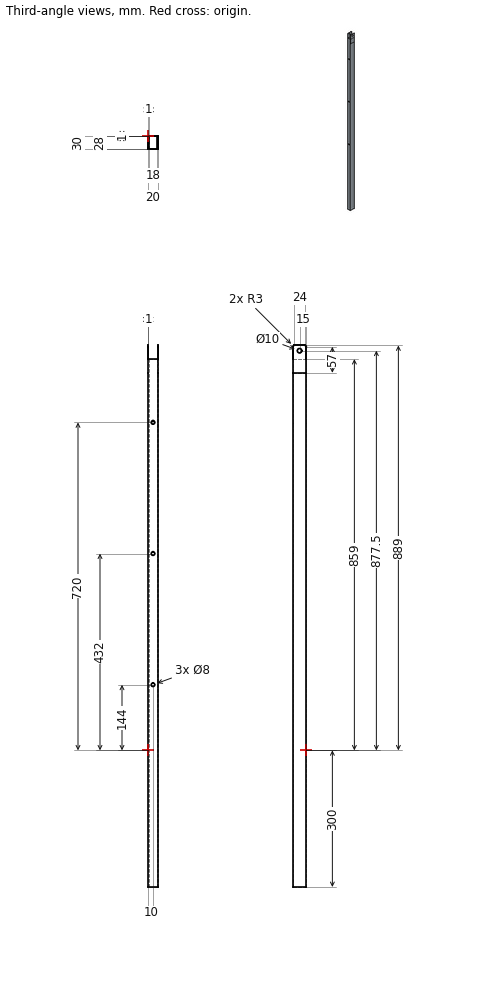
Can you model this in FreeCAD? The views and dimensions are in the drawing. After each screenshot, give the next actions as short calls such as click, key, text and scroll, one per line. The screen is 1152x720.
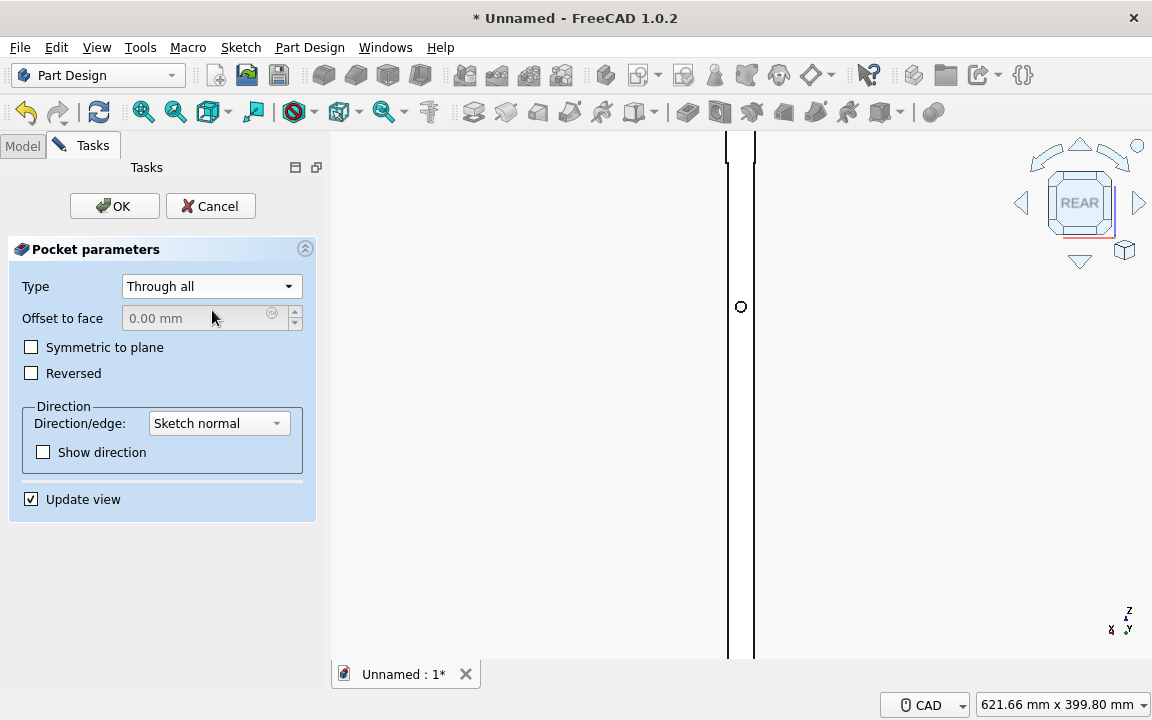
click(115, 206)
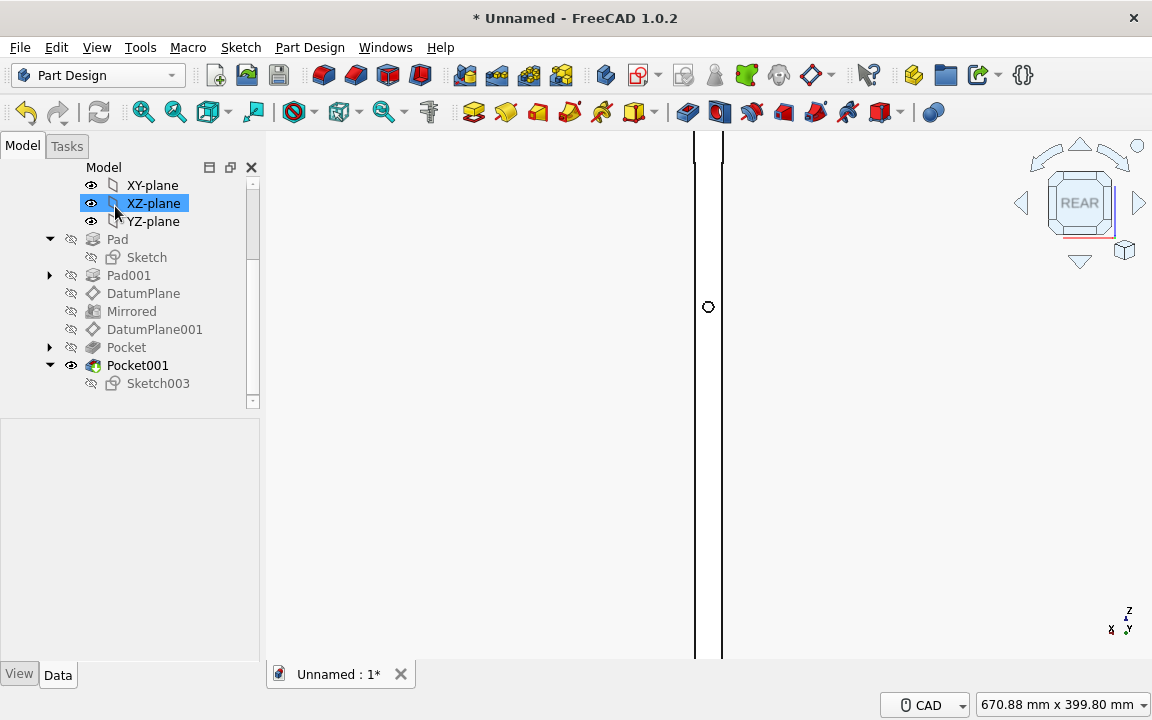
key(v)
key(f)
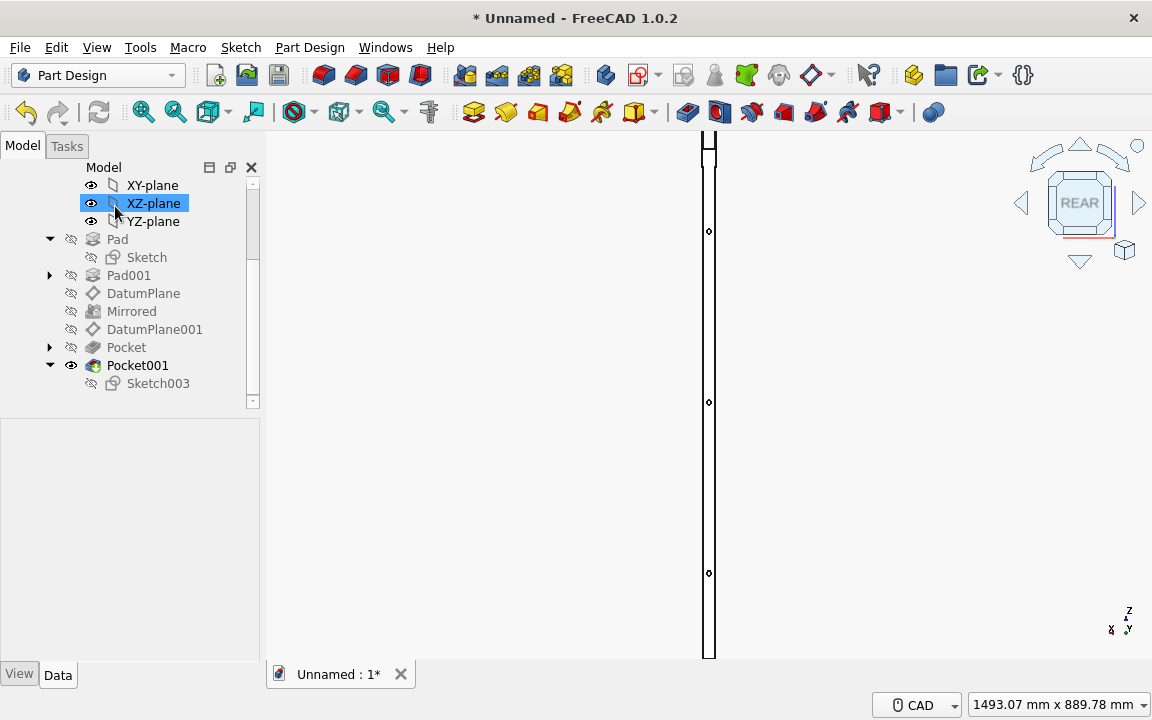
key(5)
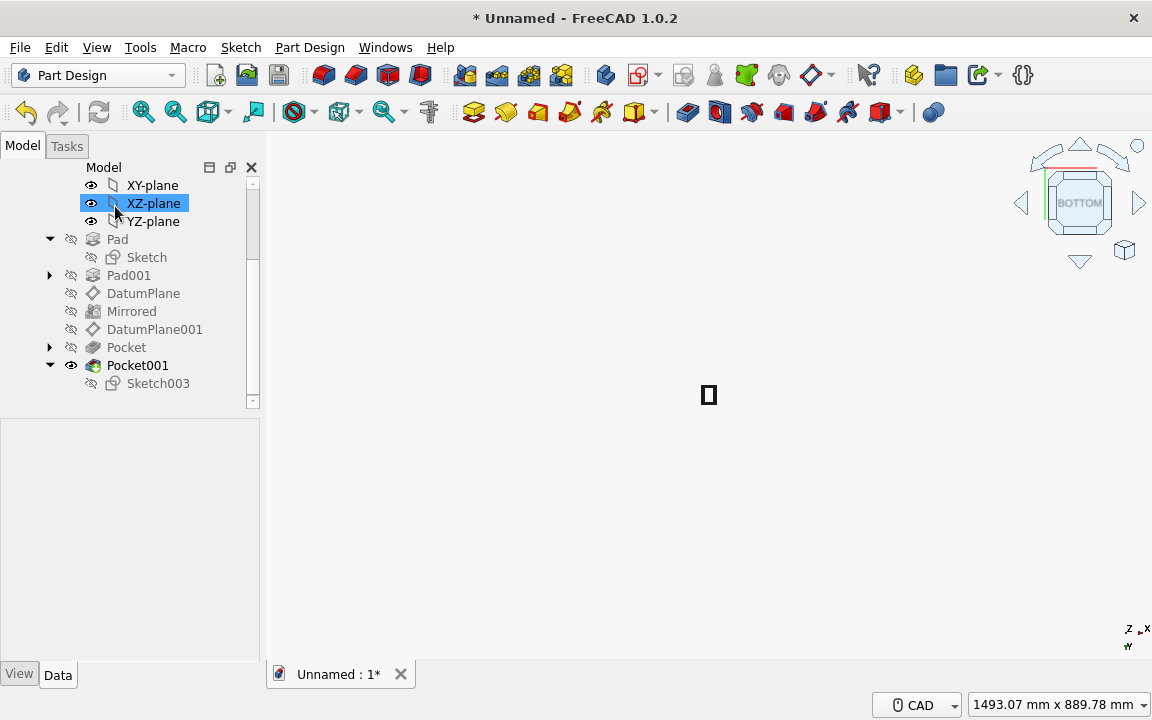
click(144, 112)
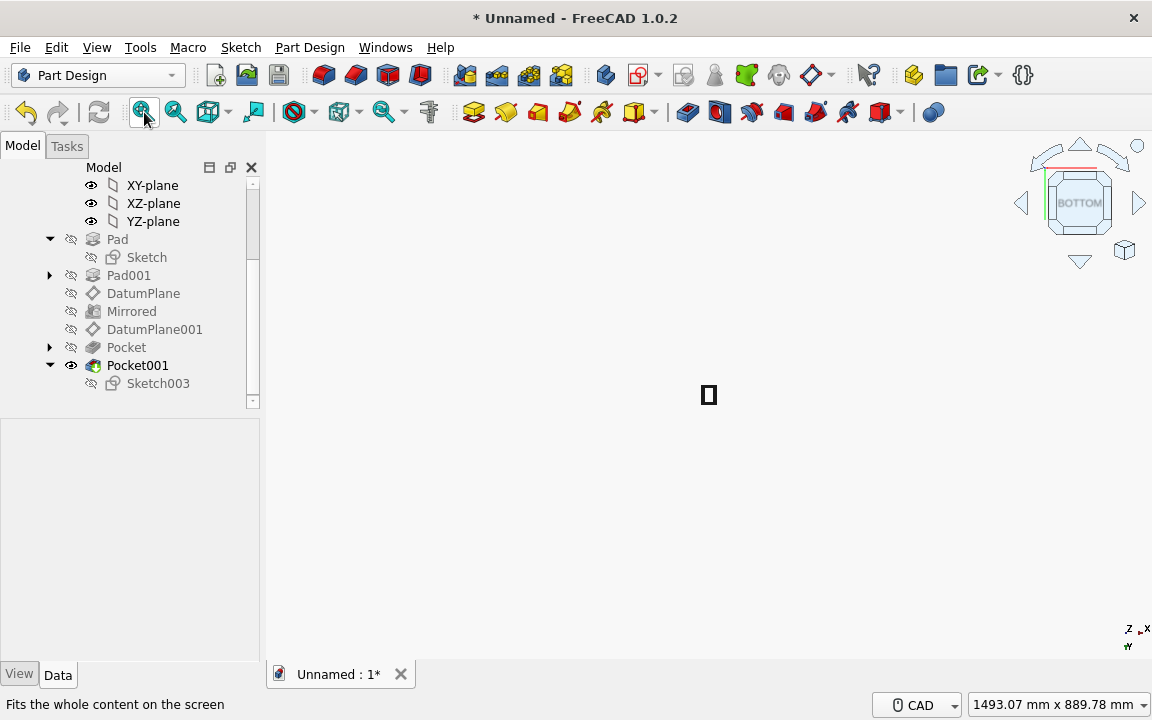
scroll(711, 403, up, 15)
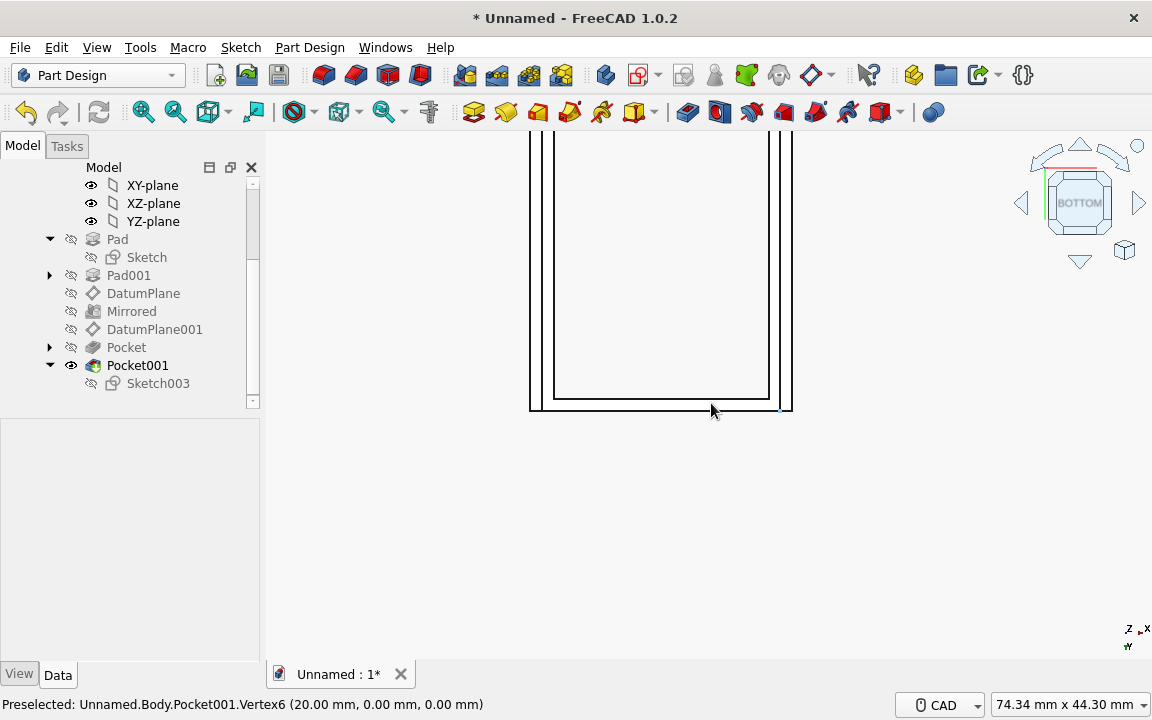
scroll(701, 402, up, 6)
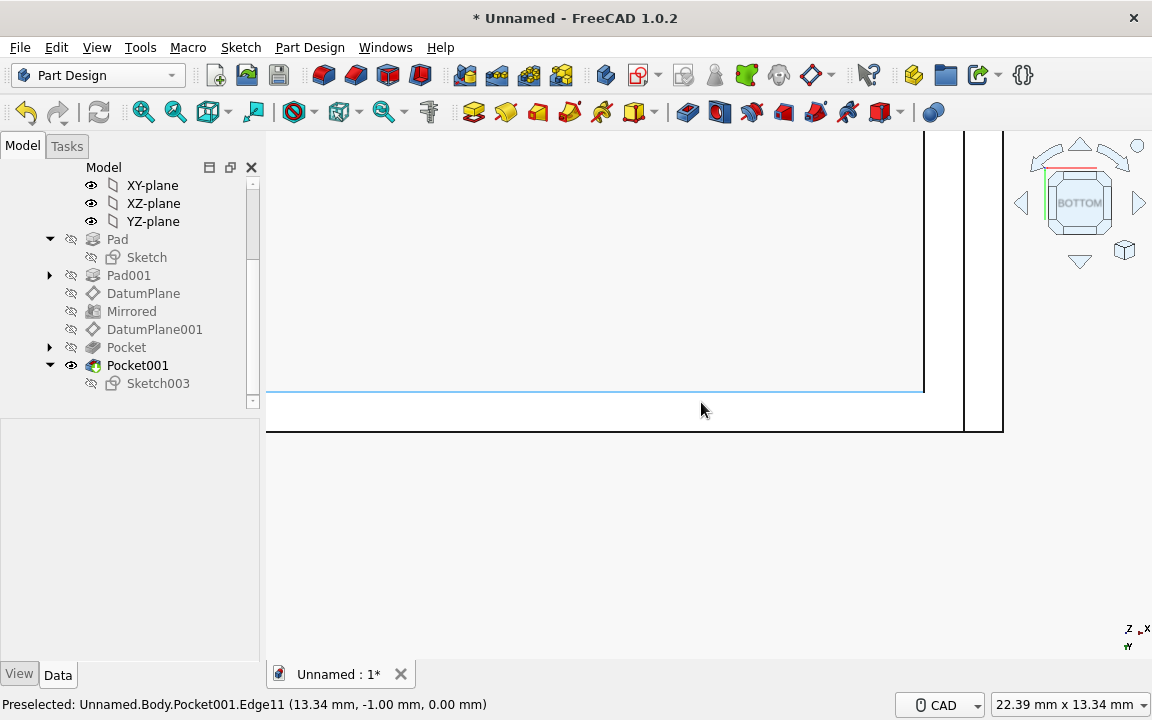
click(700, 404)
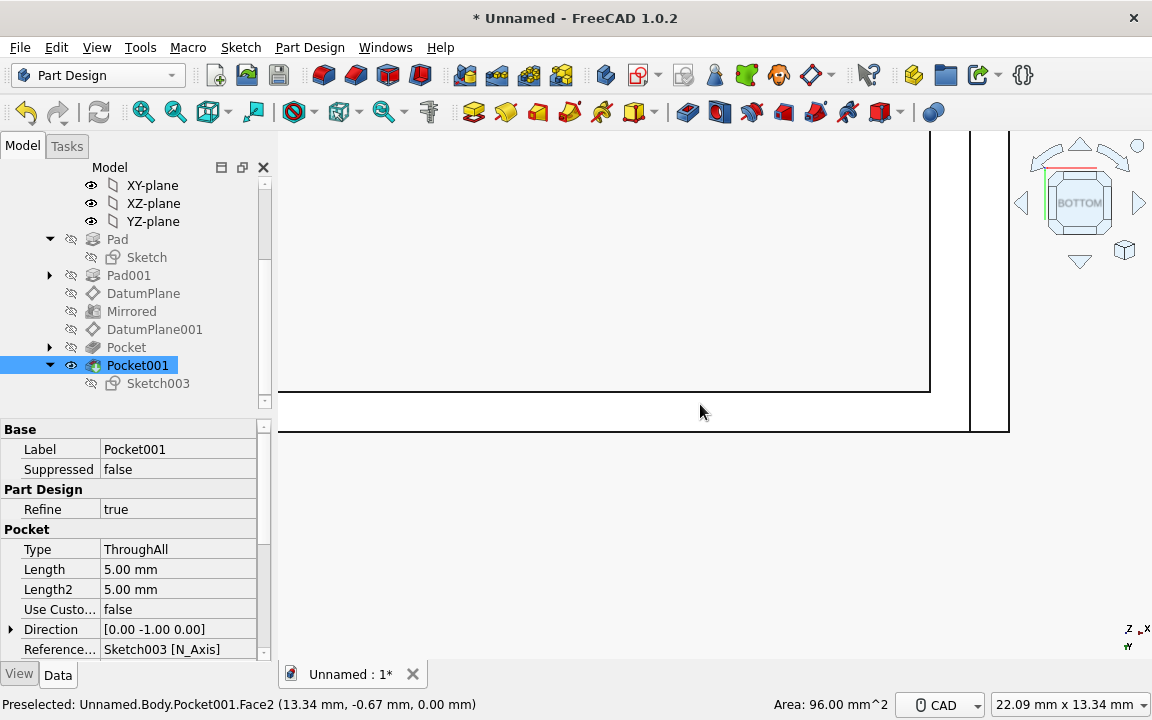
click(638, 76)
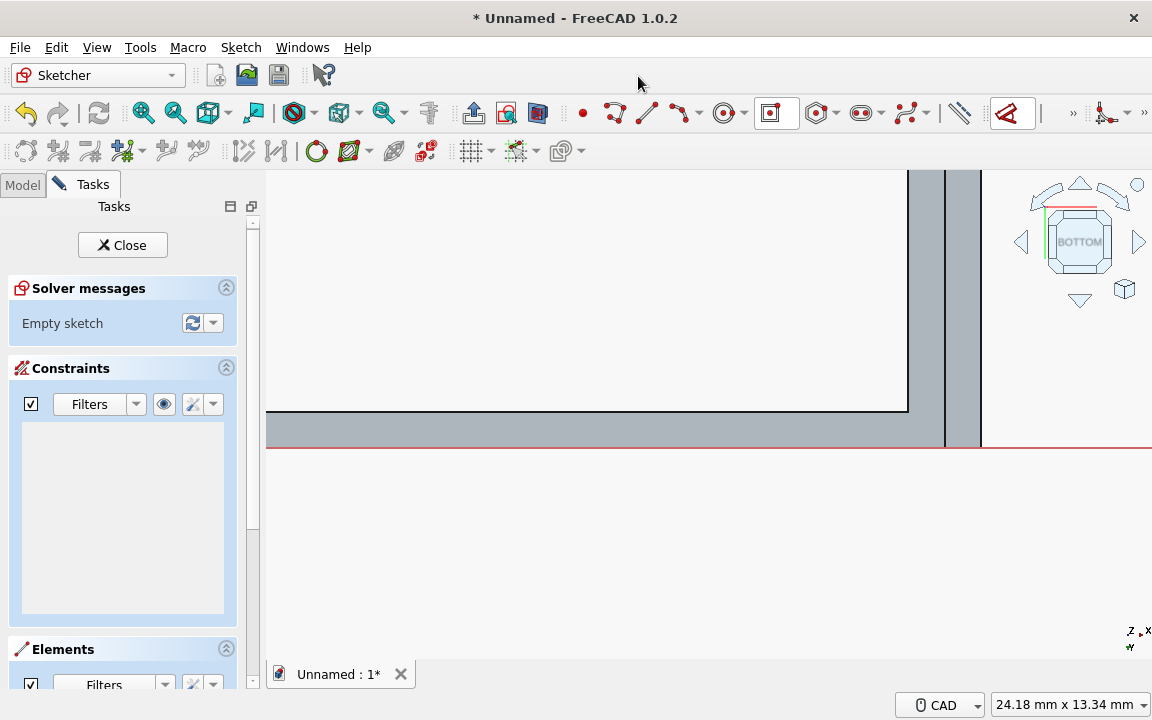
scroll(667, 631, down, 6)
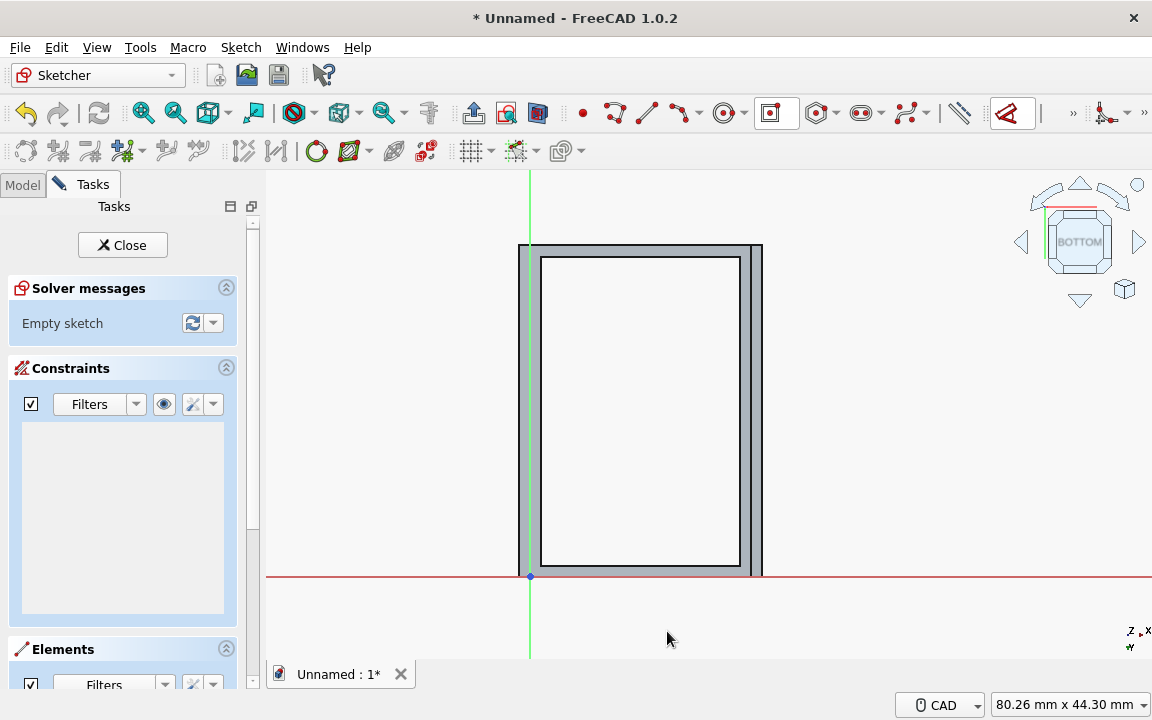
key(g)
key(r)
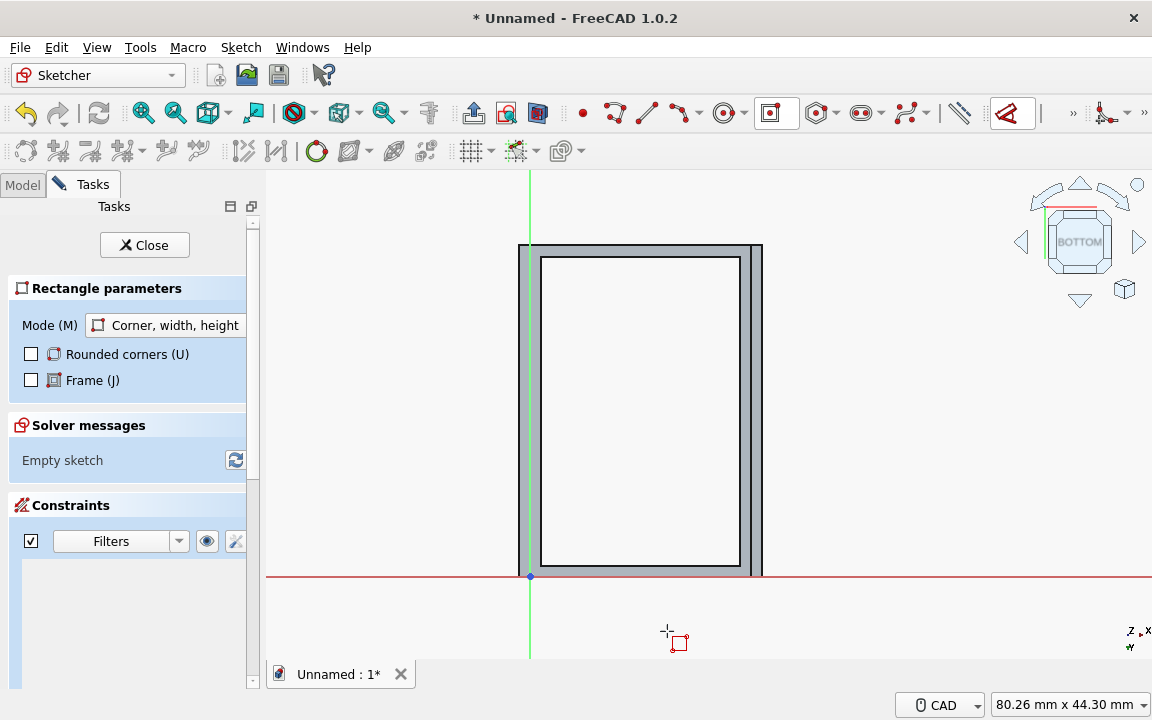
click(530, 577)
click(751, 245)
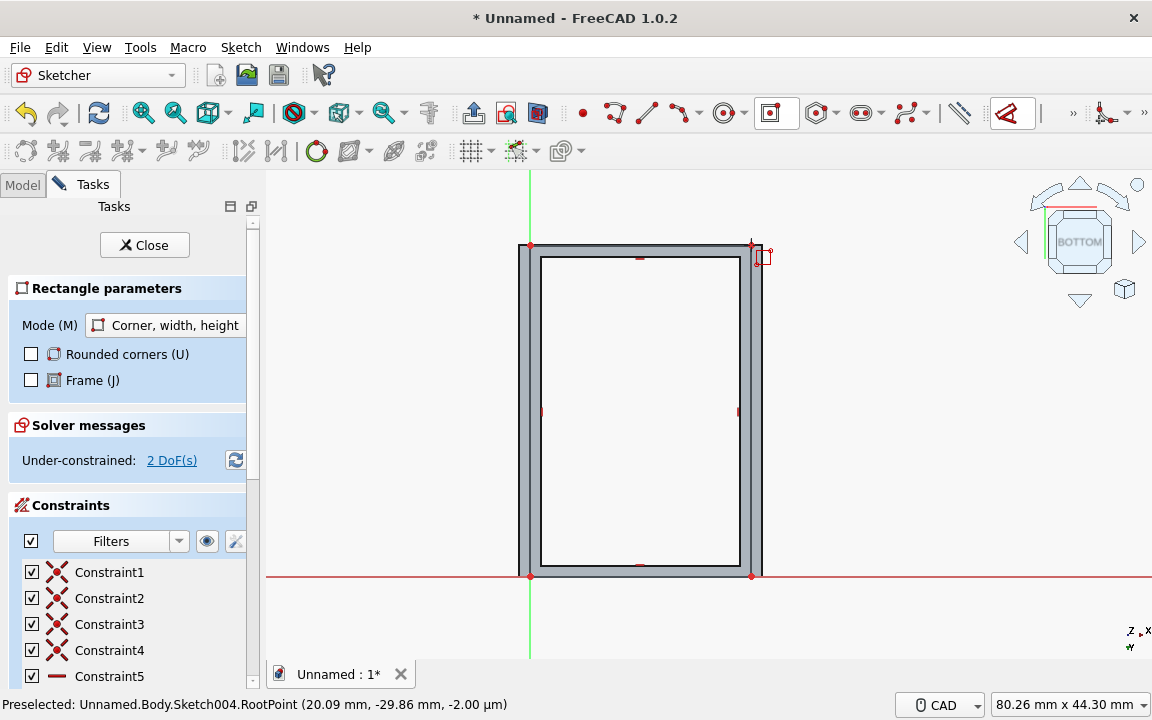
scroll(541, 257, up, 2)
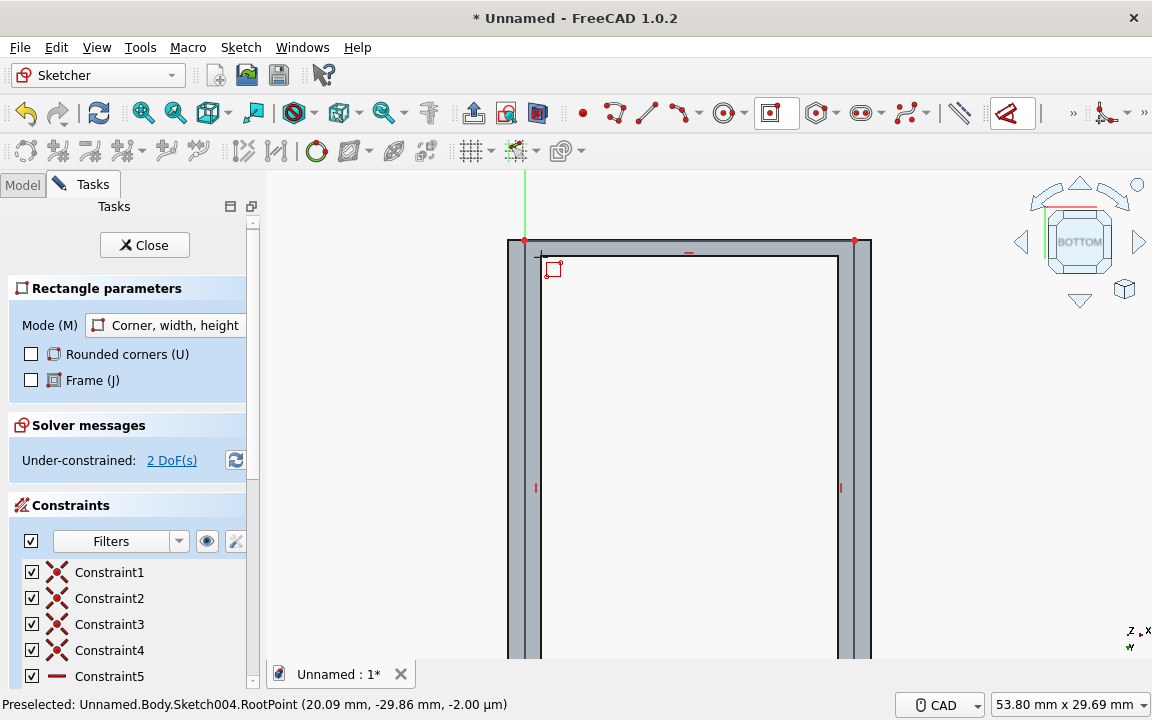
click(541, 256)